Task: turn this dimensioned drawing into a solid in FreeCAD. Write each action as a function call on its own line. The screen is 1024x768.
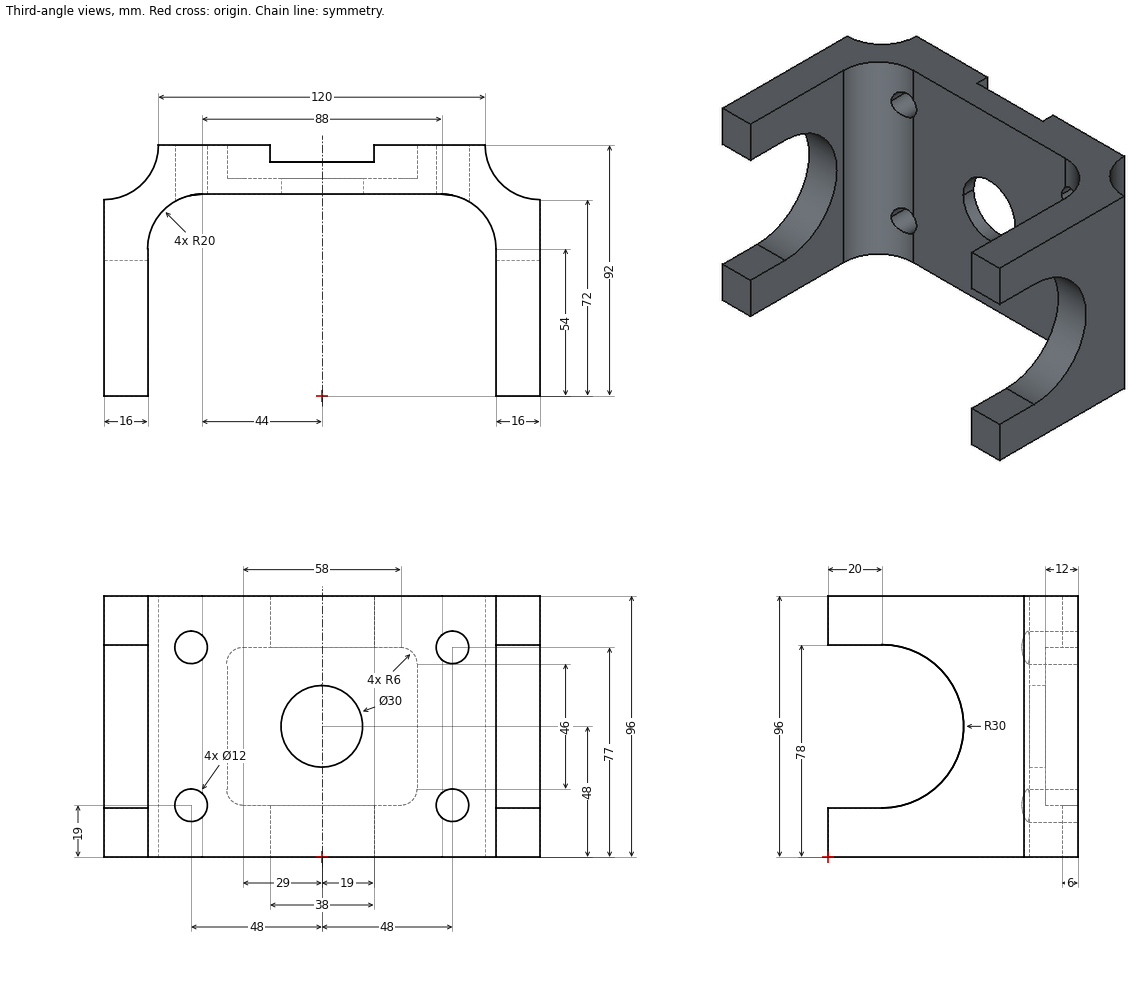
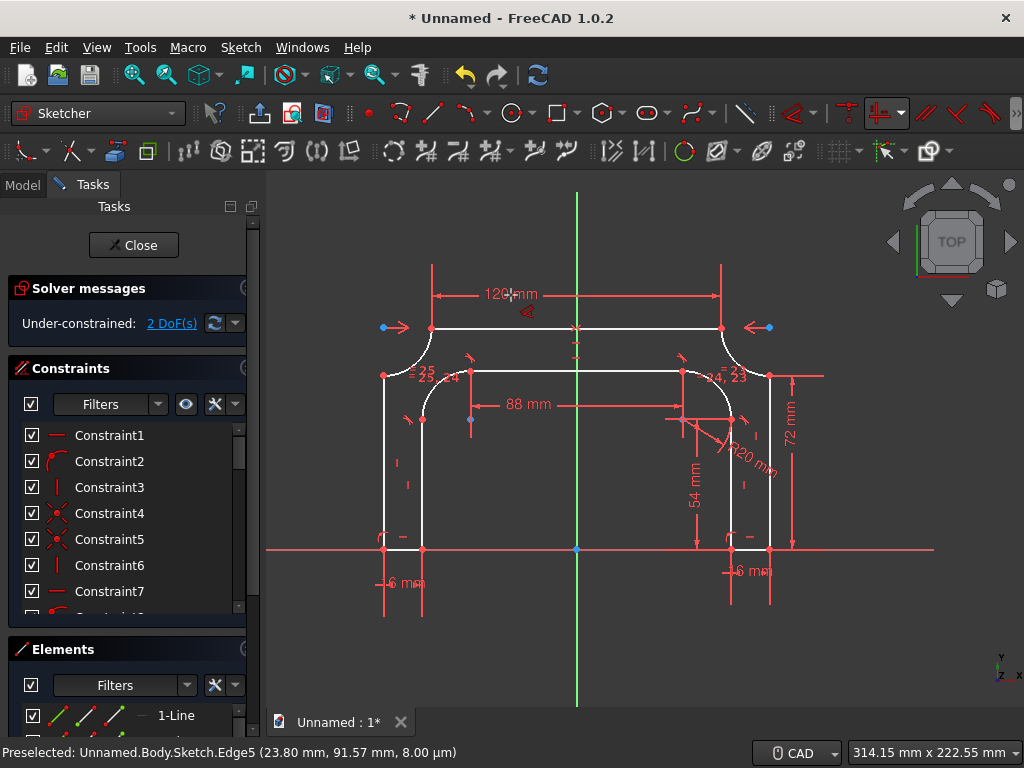
click(471, 371)
click(524, 584)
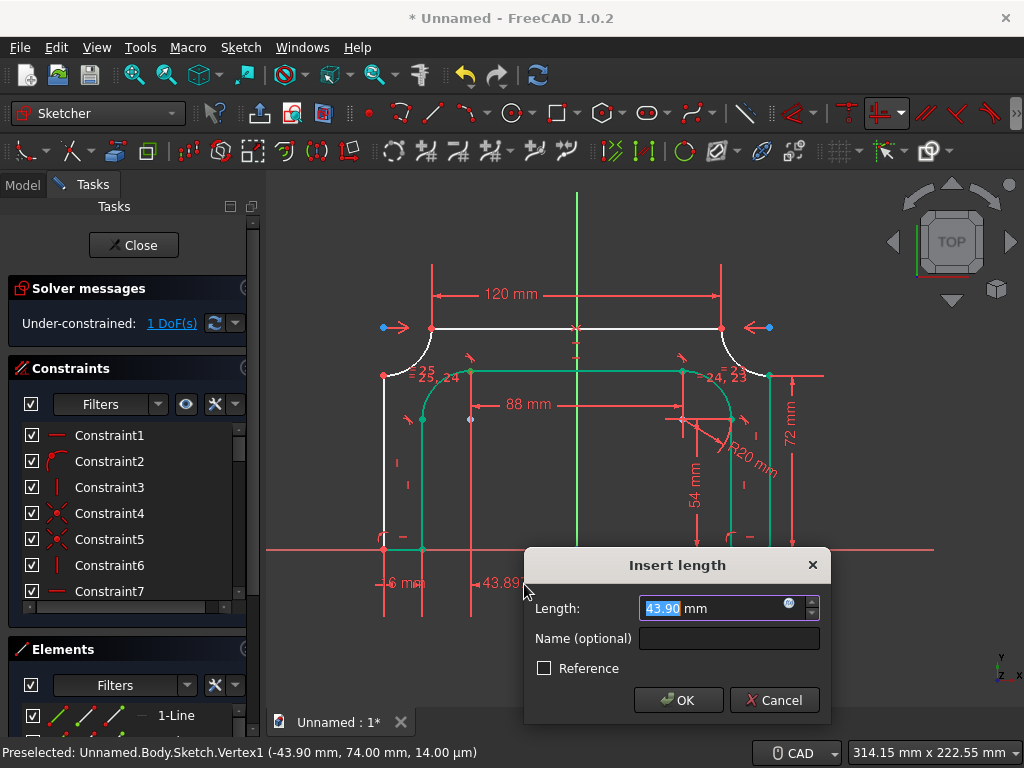
text(44)
key(Return)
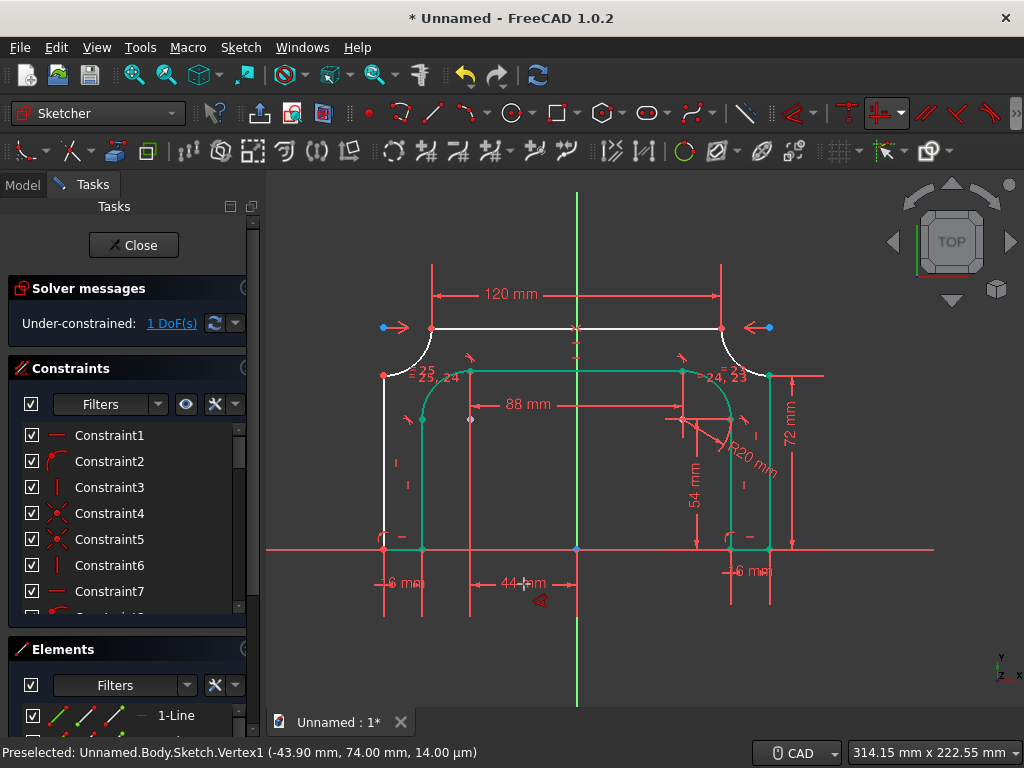
click(721, 329)
click(755, 388)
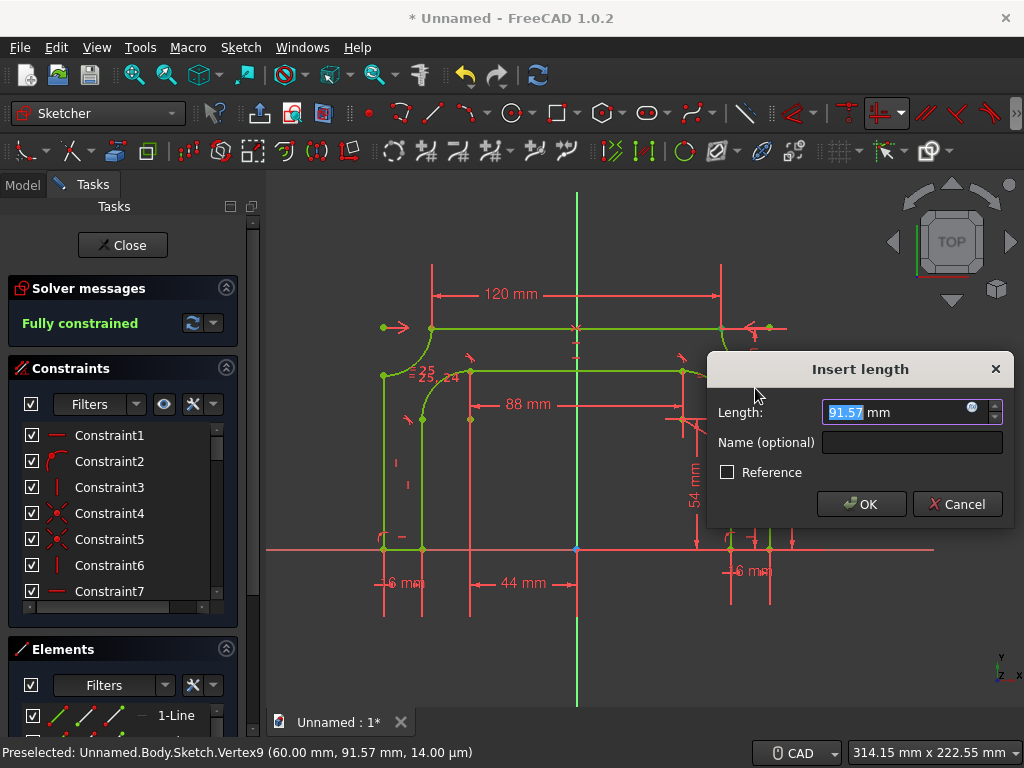
text(92)
key(Return)
key(Escape)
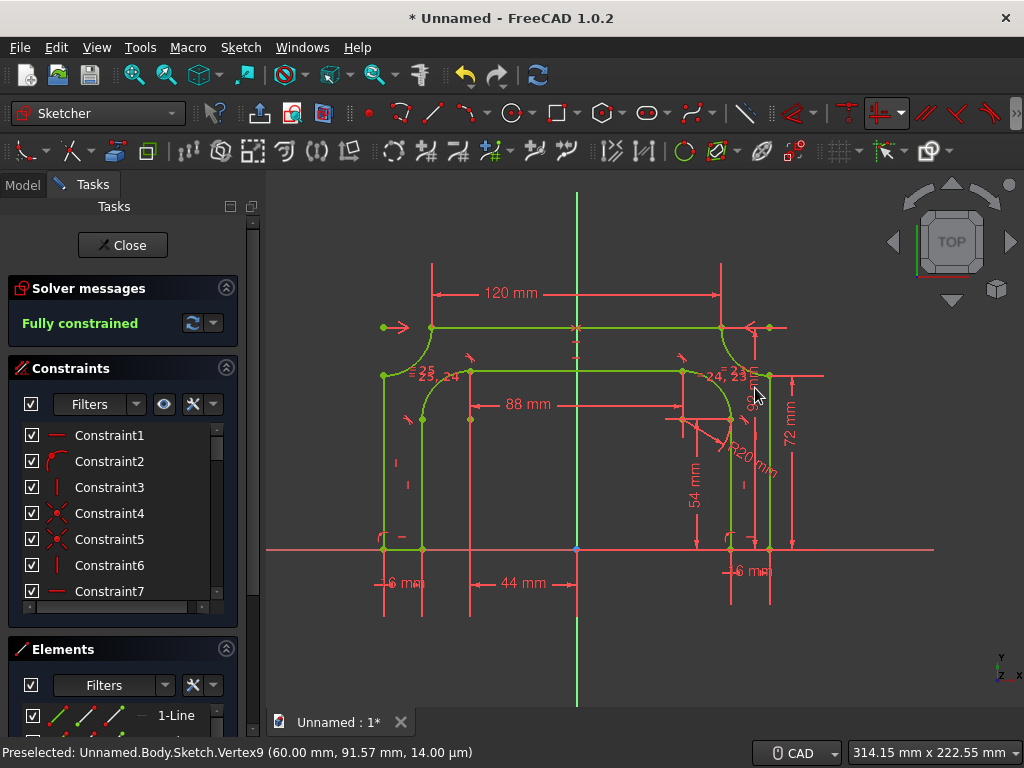
click(123, 245)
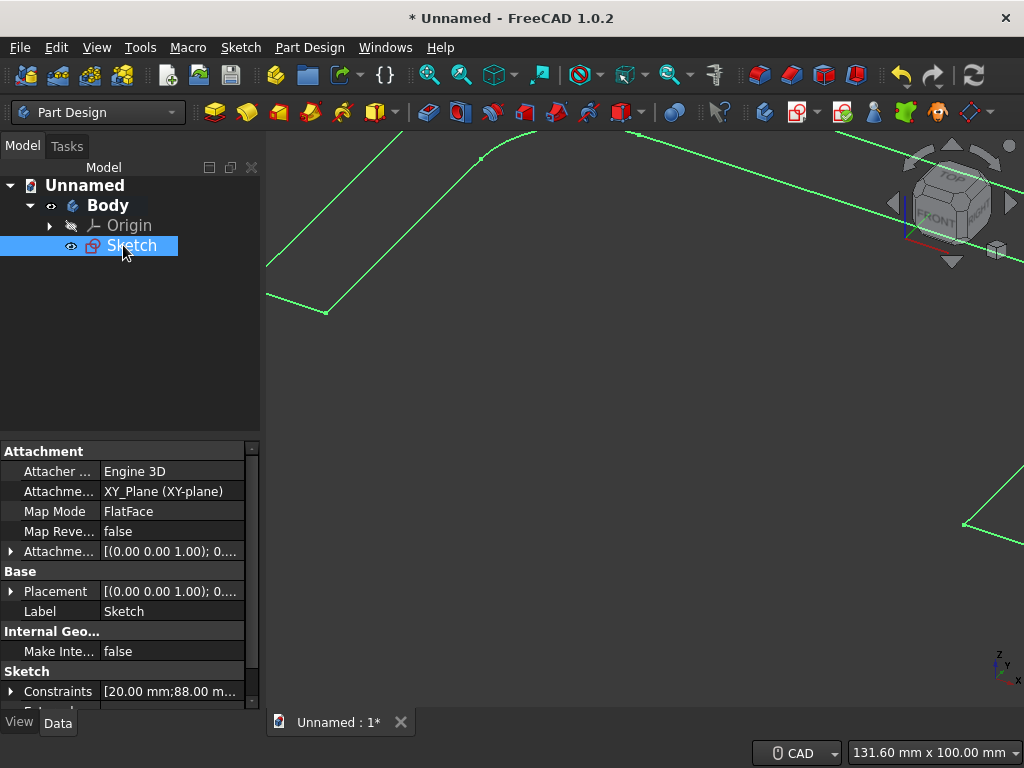
click(216, 112)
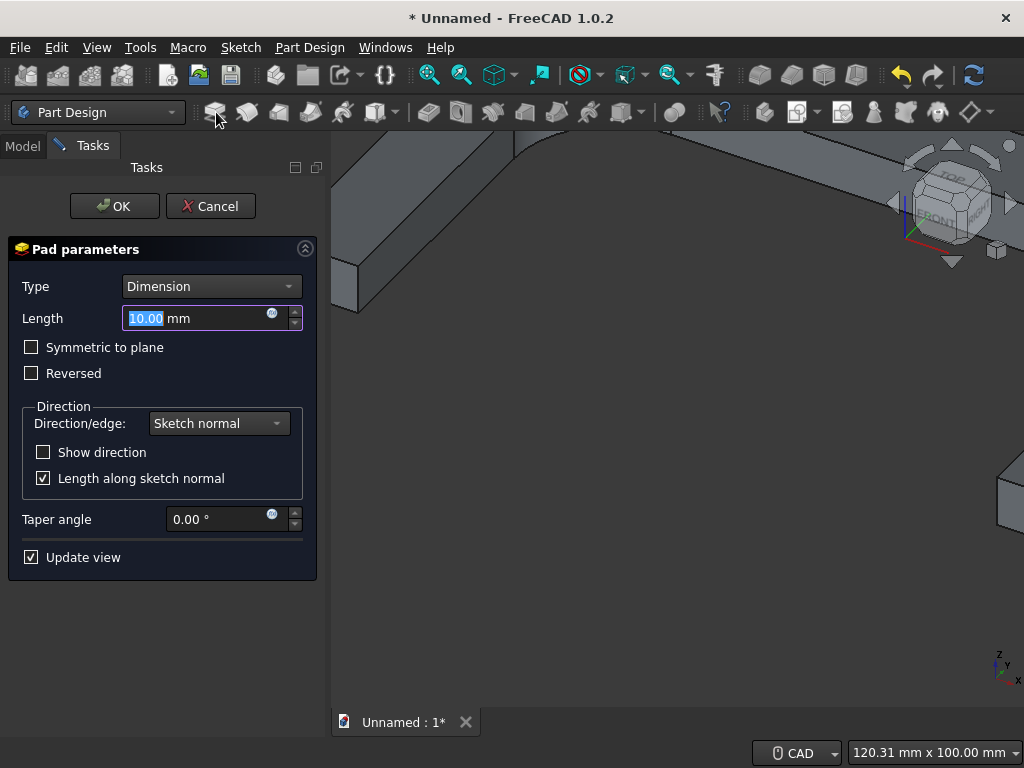
text(96)
key(Tab)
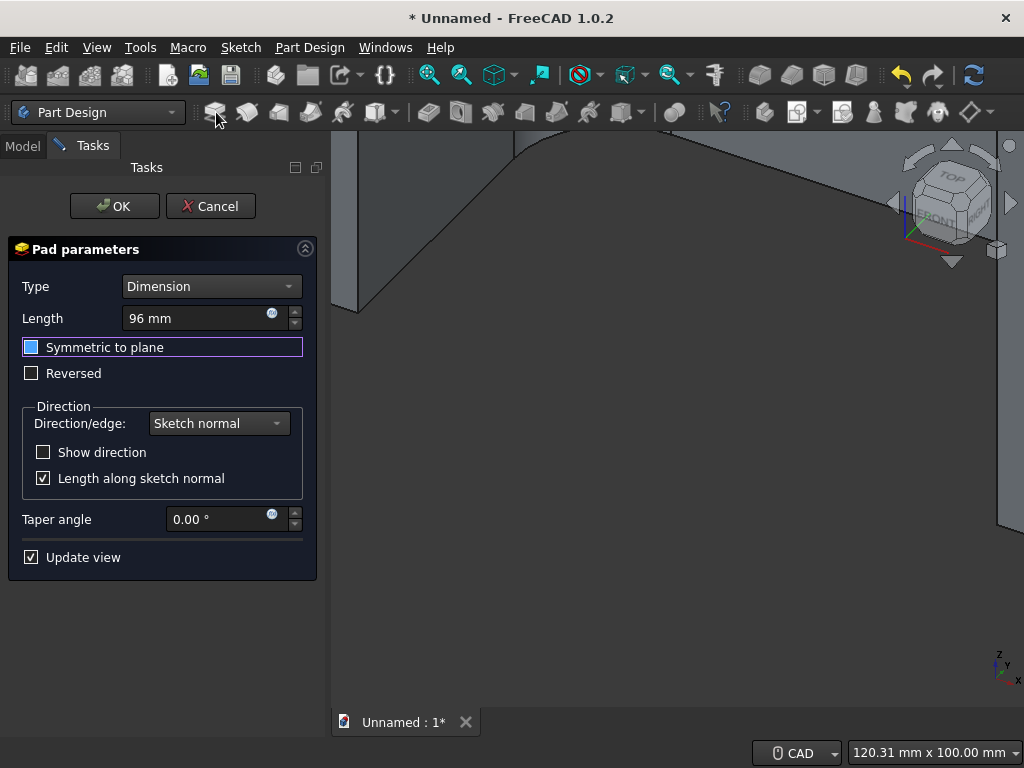
click(115, 206)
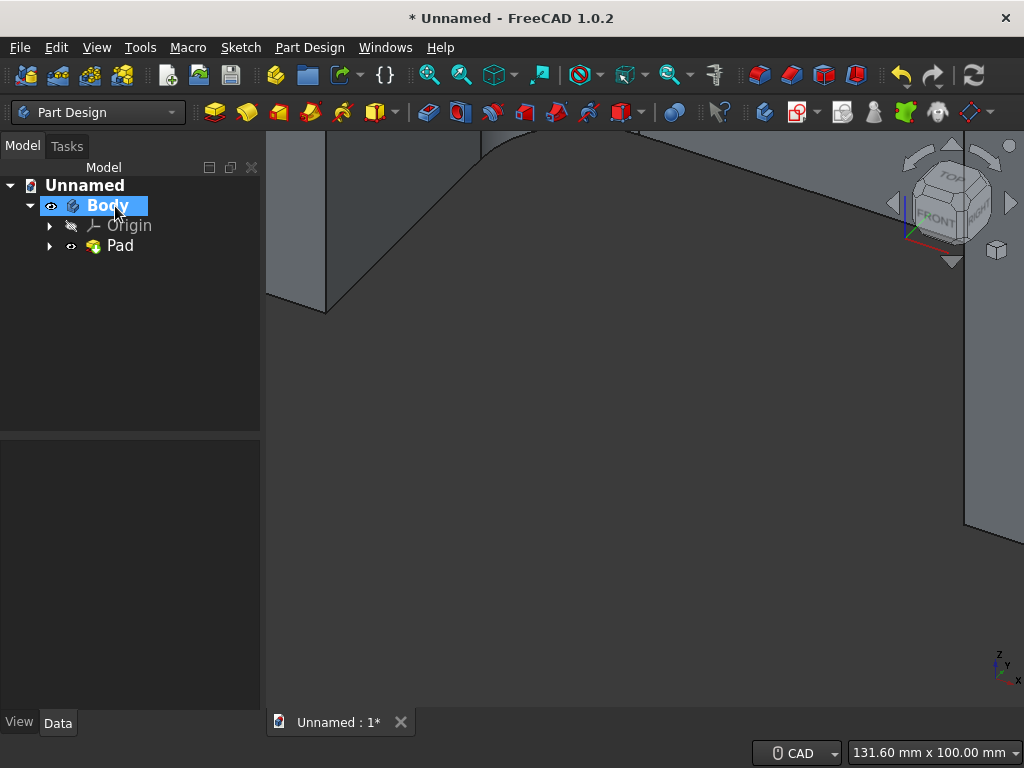
click(430, 76)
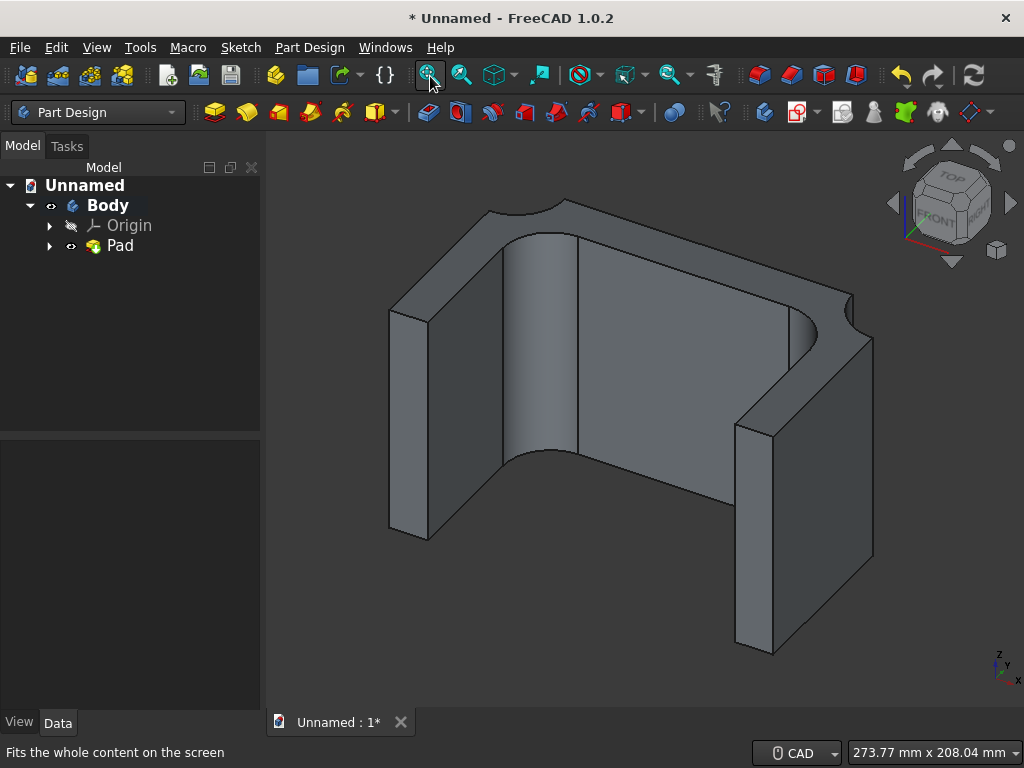
click(823, 495)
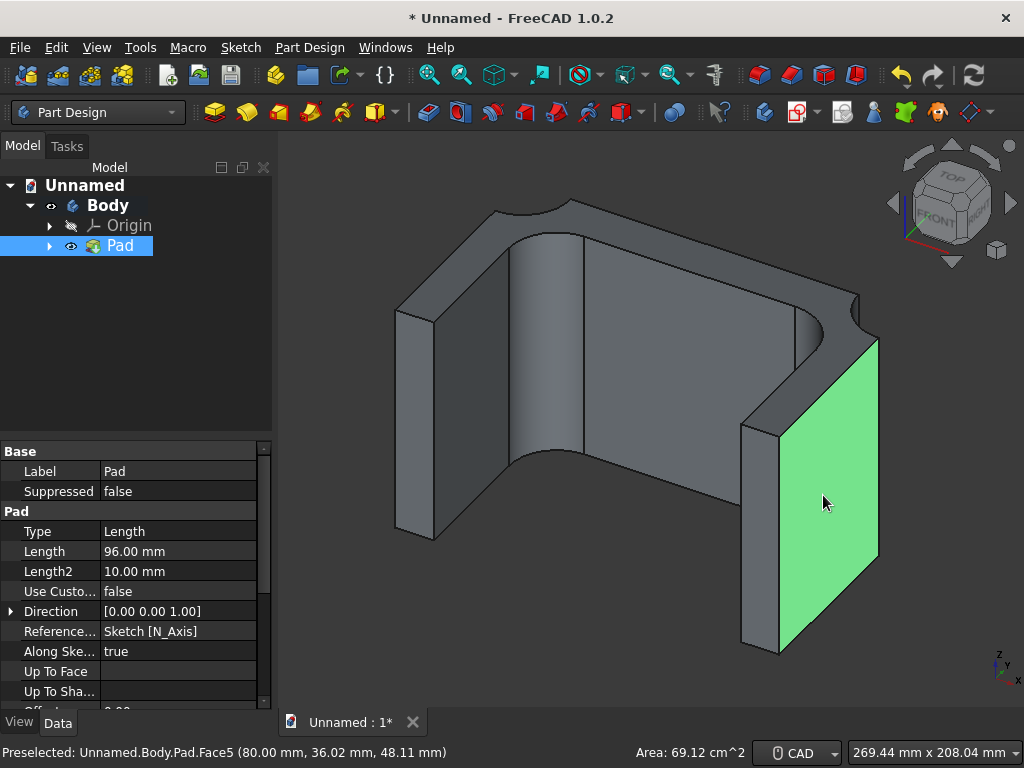
click(798, 112)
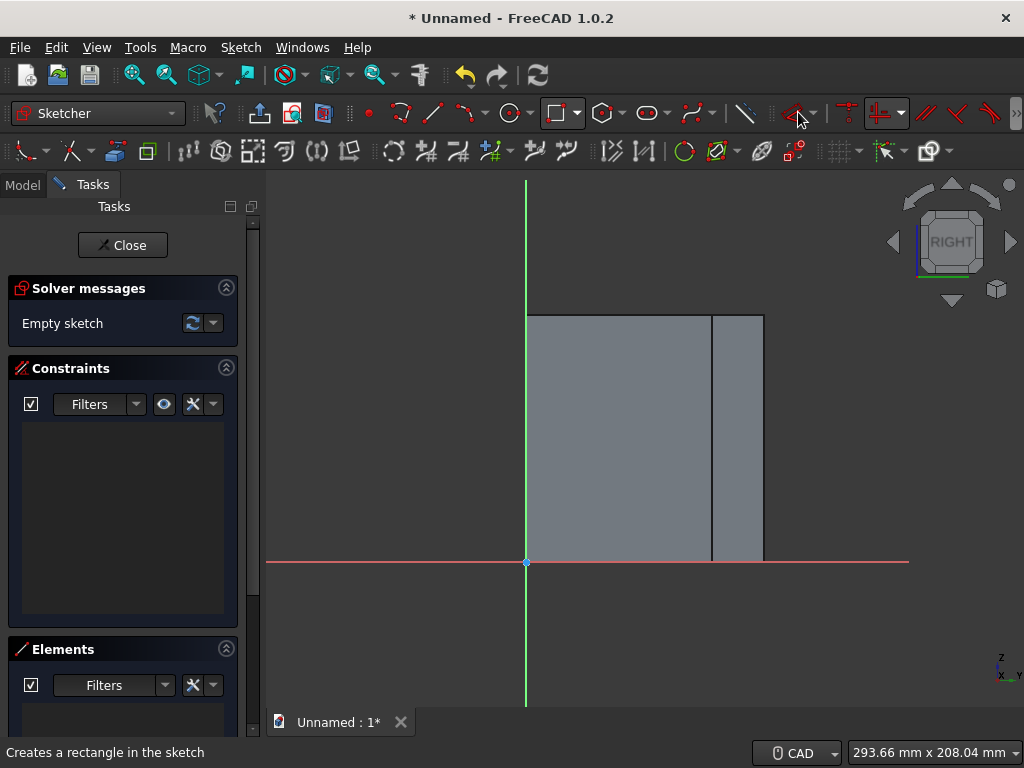
scroll(608, 490, up, 3)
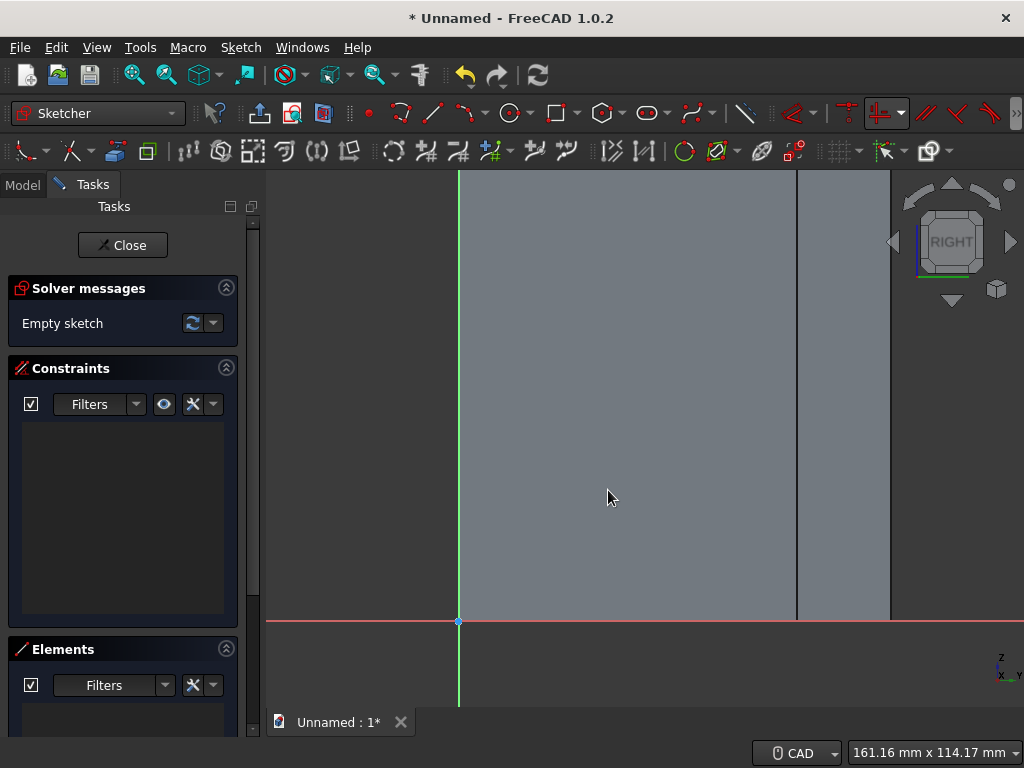
click(402, 114)